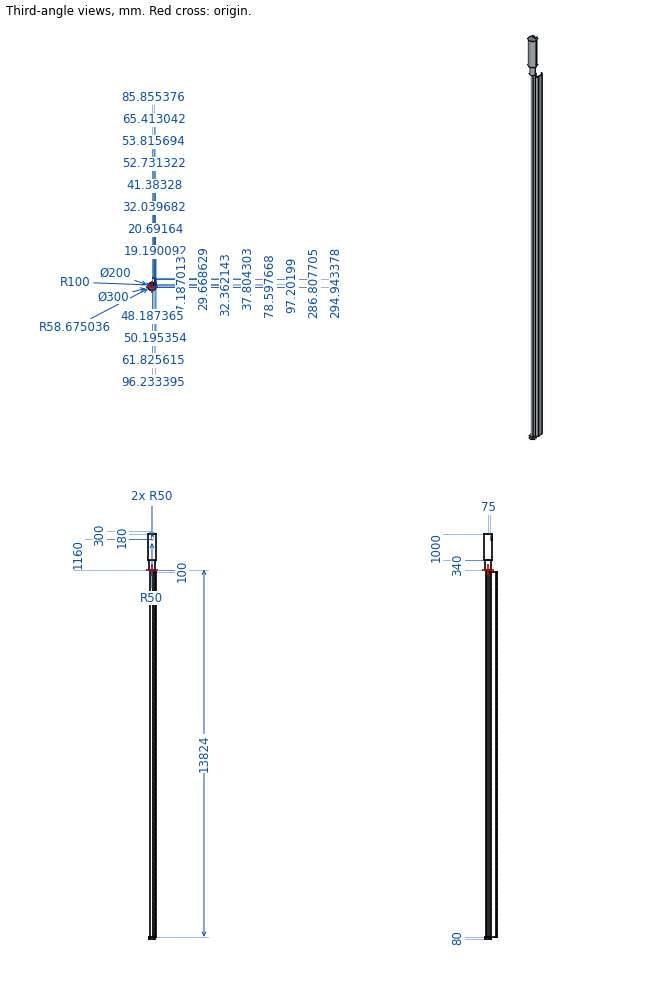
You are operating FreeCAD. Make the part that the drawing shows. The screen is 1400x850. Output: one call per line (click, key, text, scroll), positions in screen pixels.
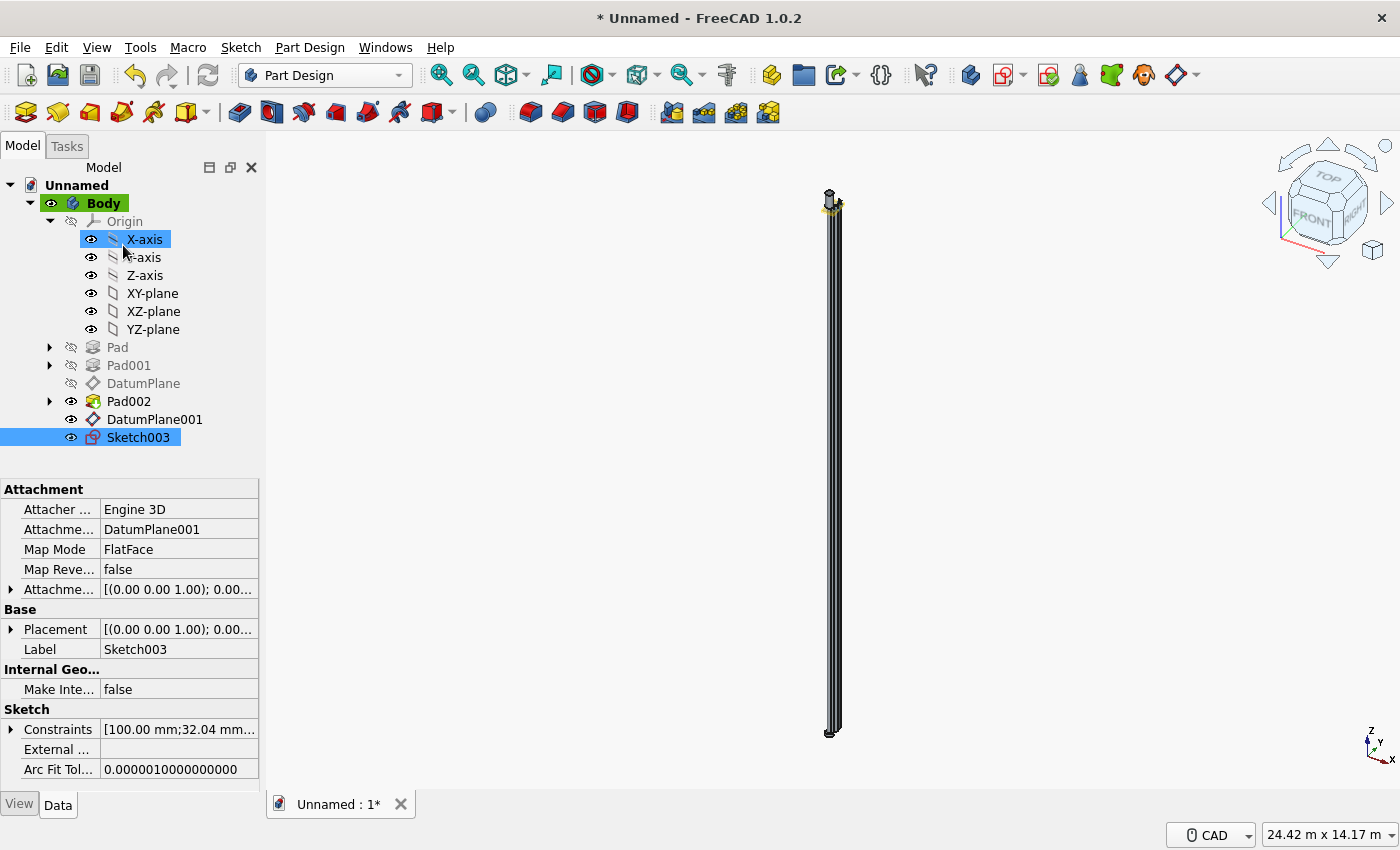
click(240, 112)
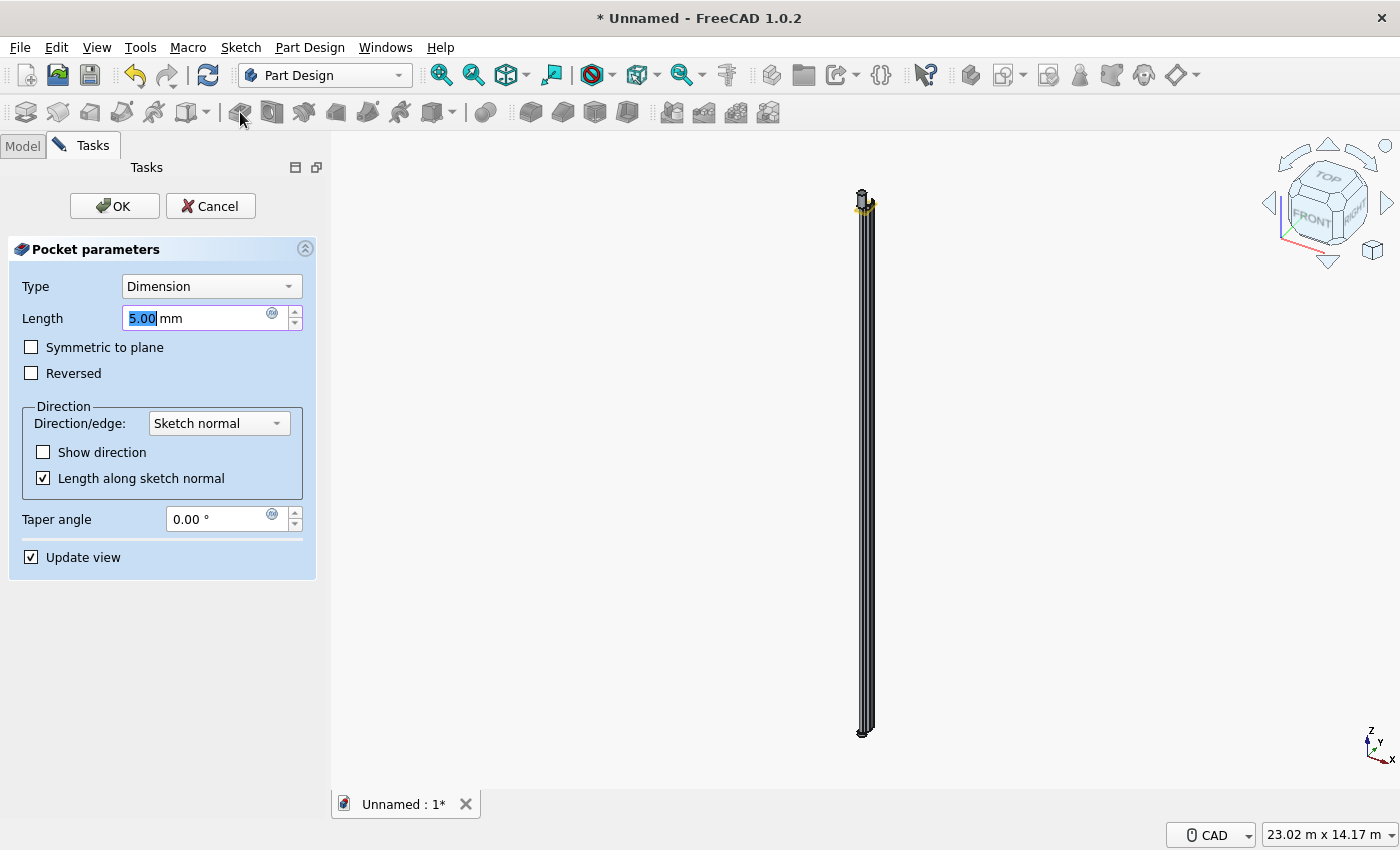
text(100)
key(Tab)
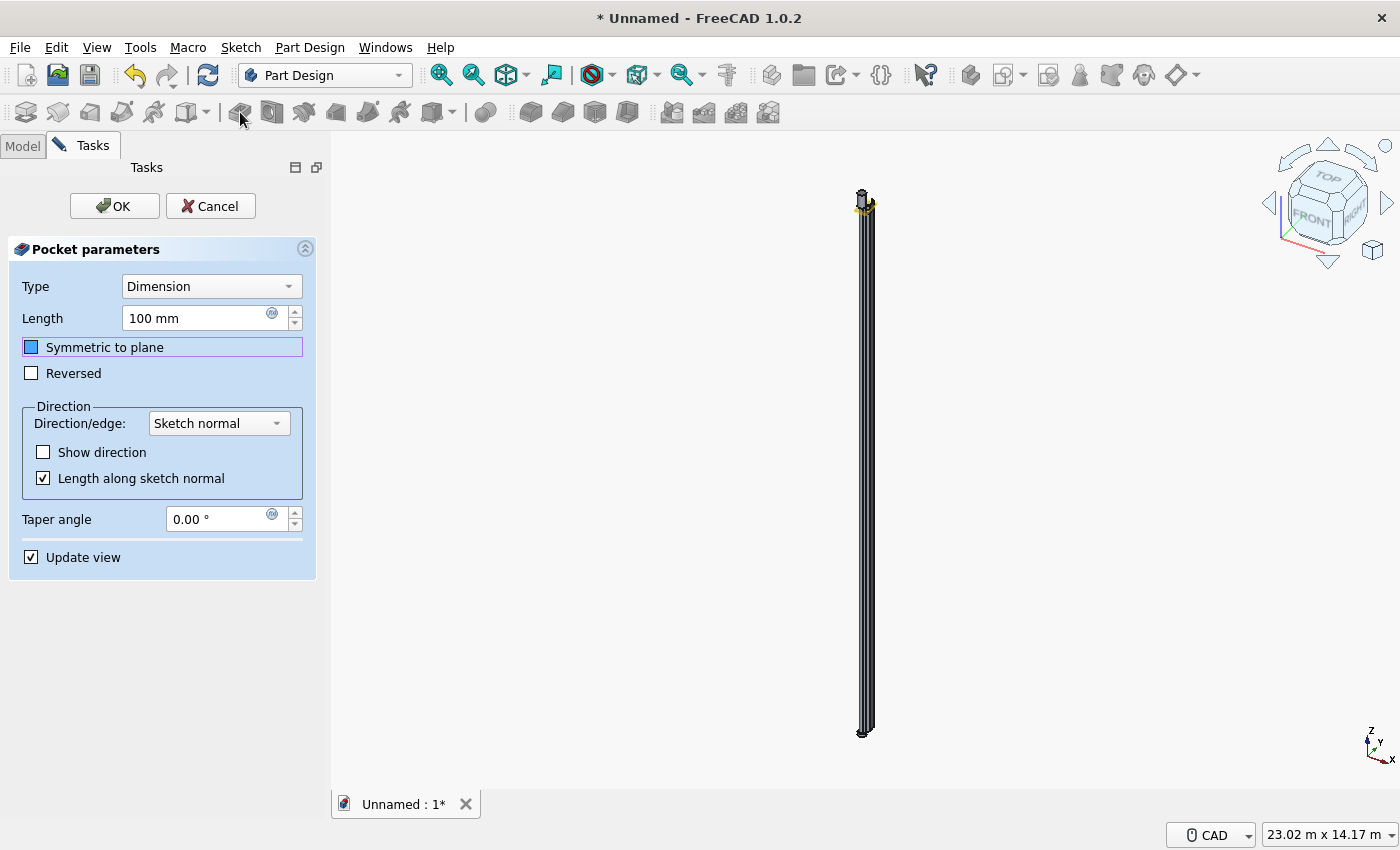
click(30, 373)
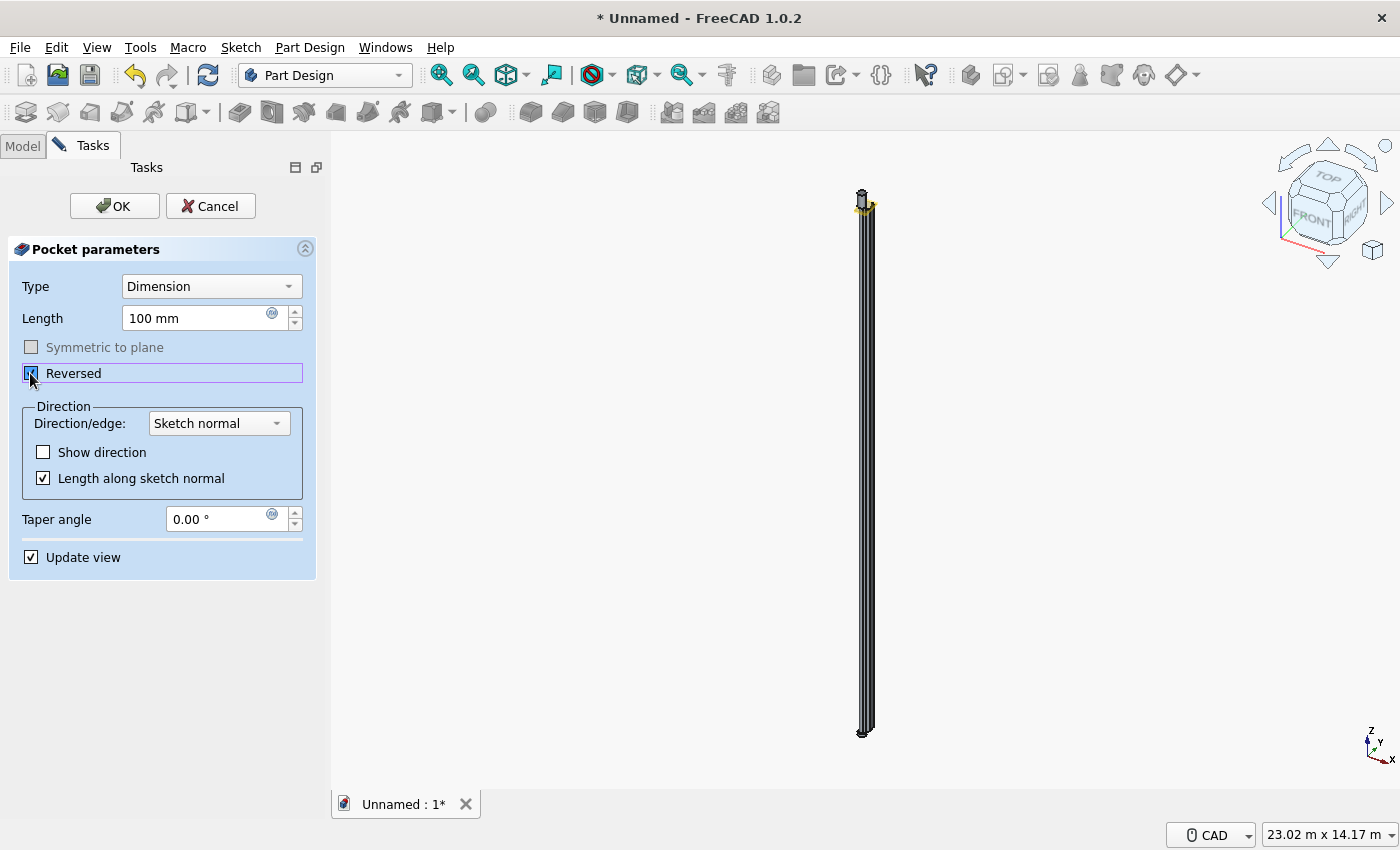
click(115, 206)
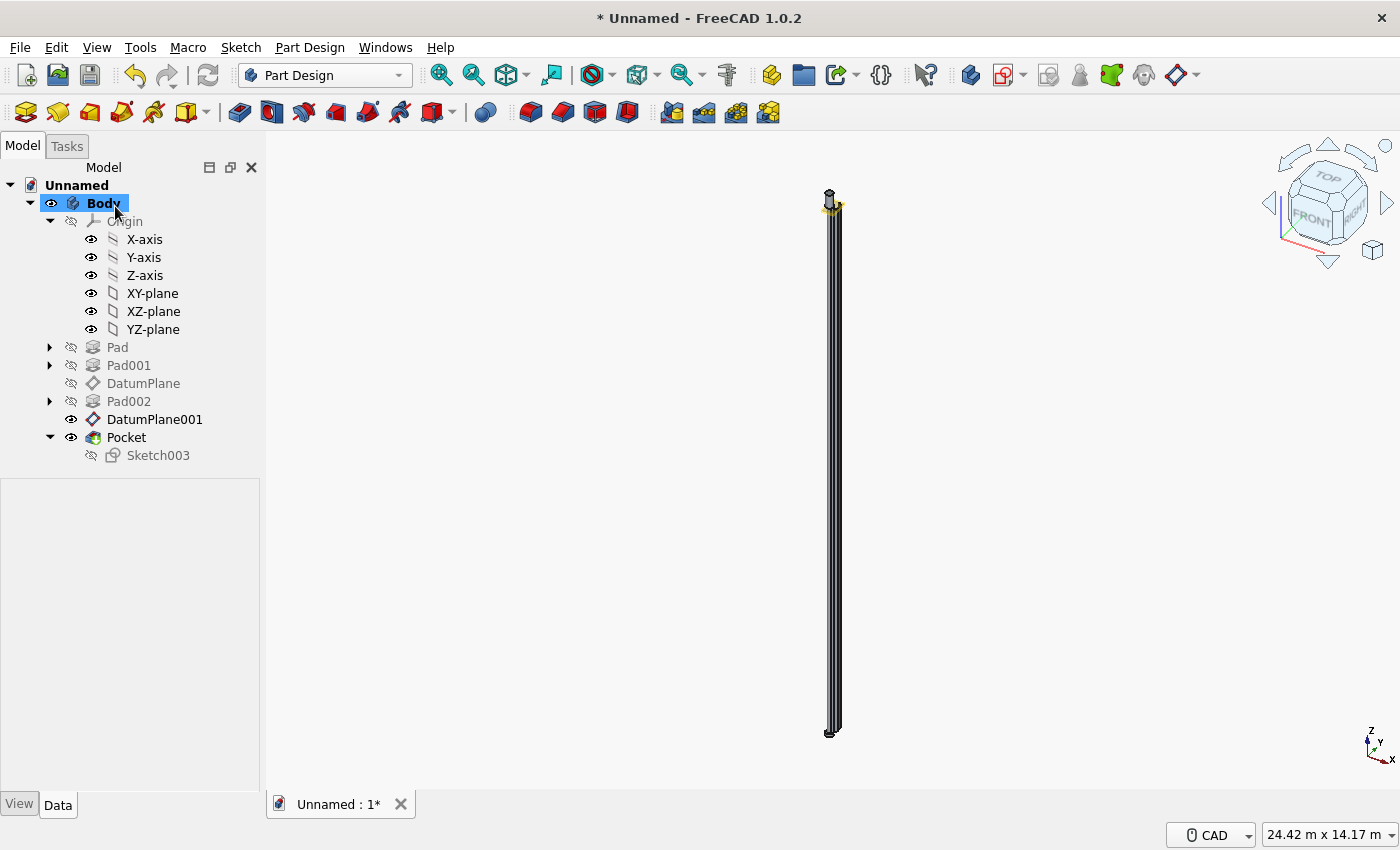
click(116, 419)
key(space)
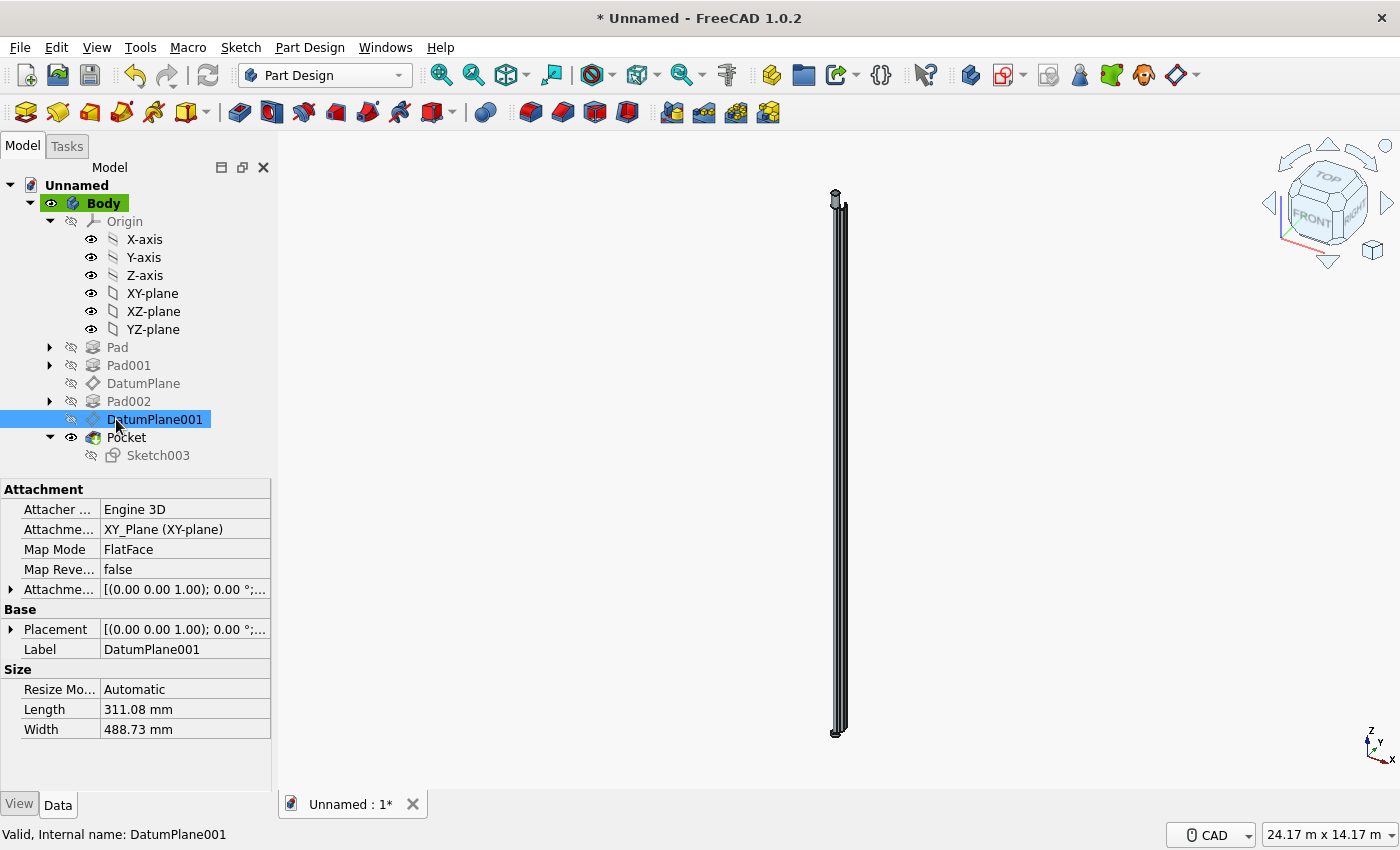
scroll(835, 192, up, 5)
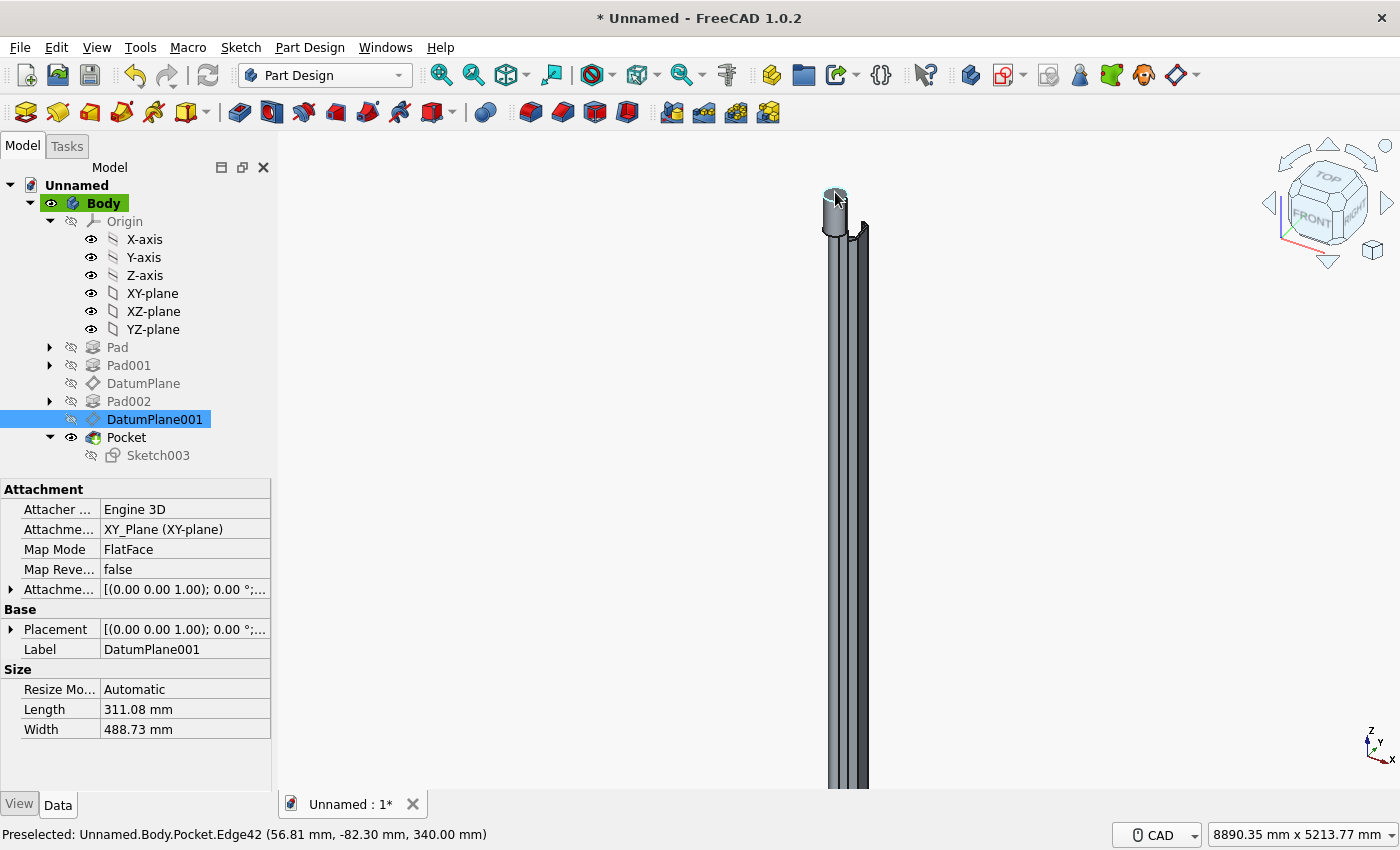
click(834, 191)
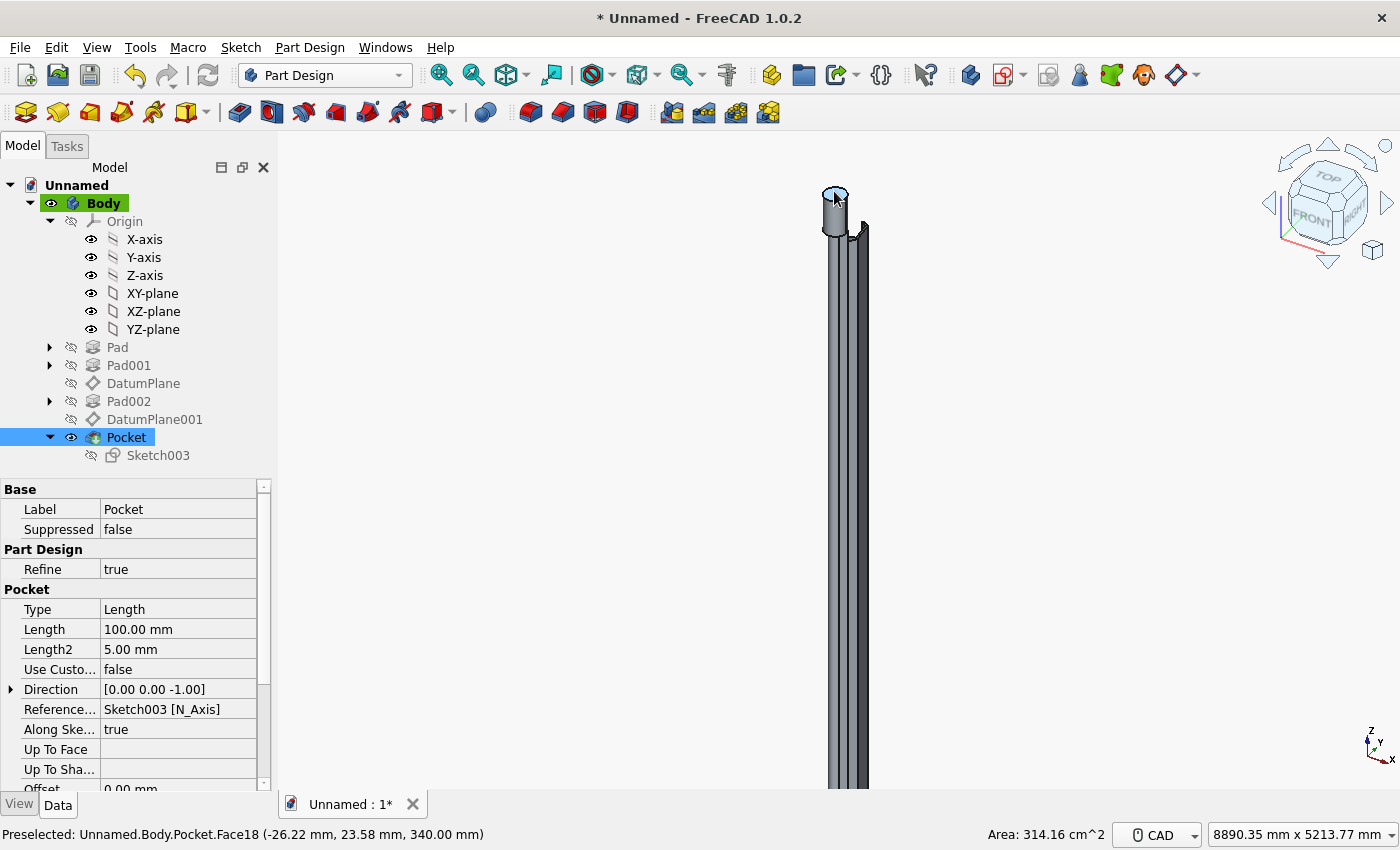
click(1004, 76)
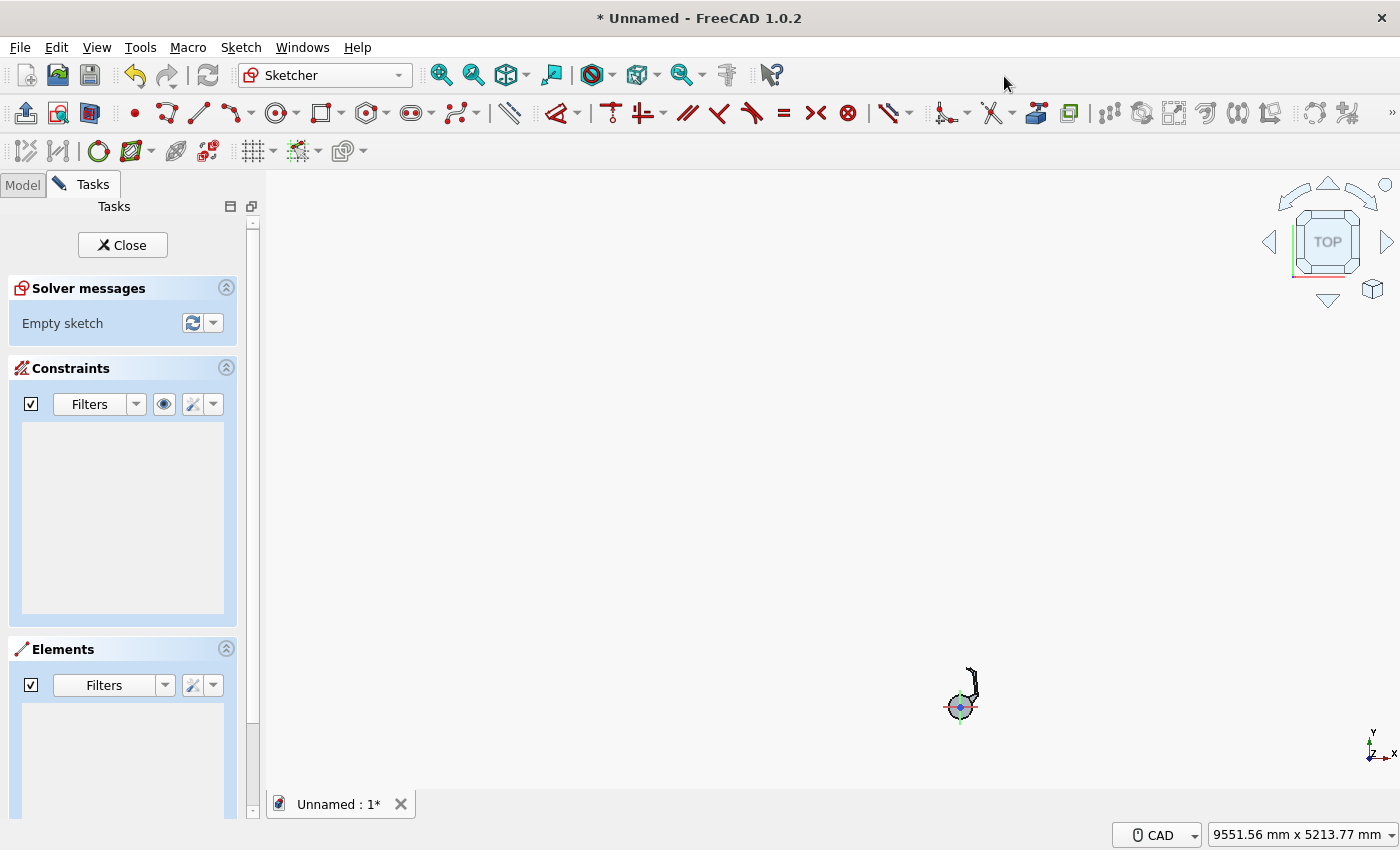
scroll(980, 730, up, 12)